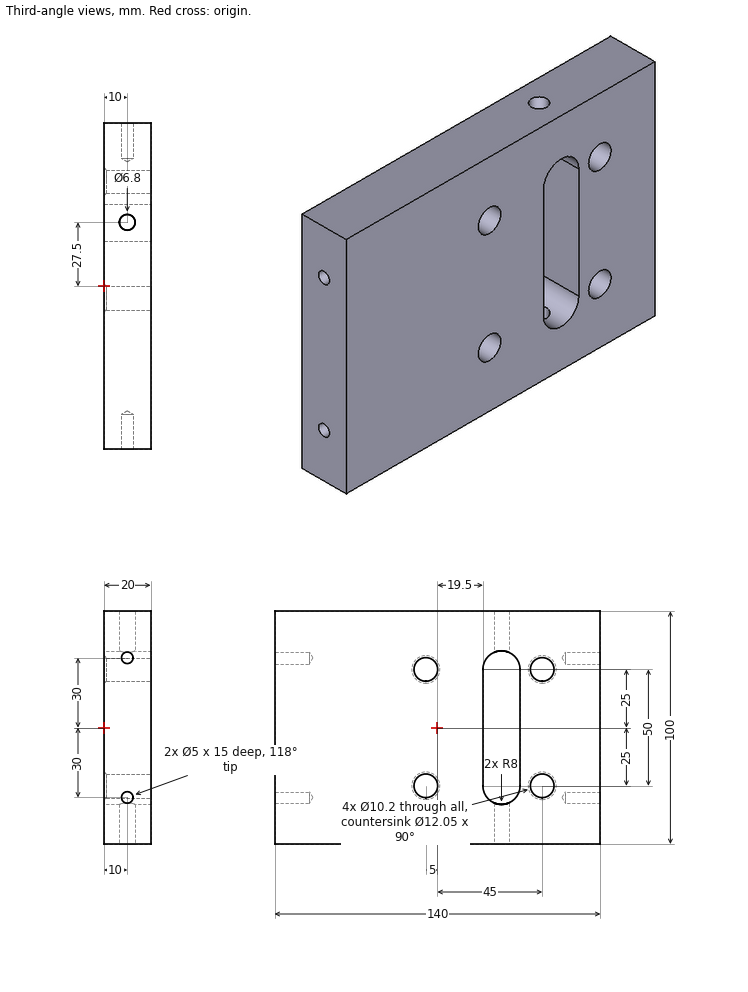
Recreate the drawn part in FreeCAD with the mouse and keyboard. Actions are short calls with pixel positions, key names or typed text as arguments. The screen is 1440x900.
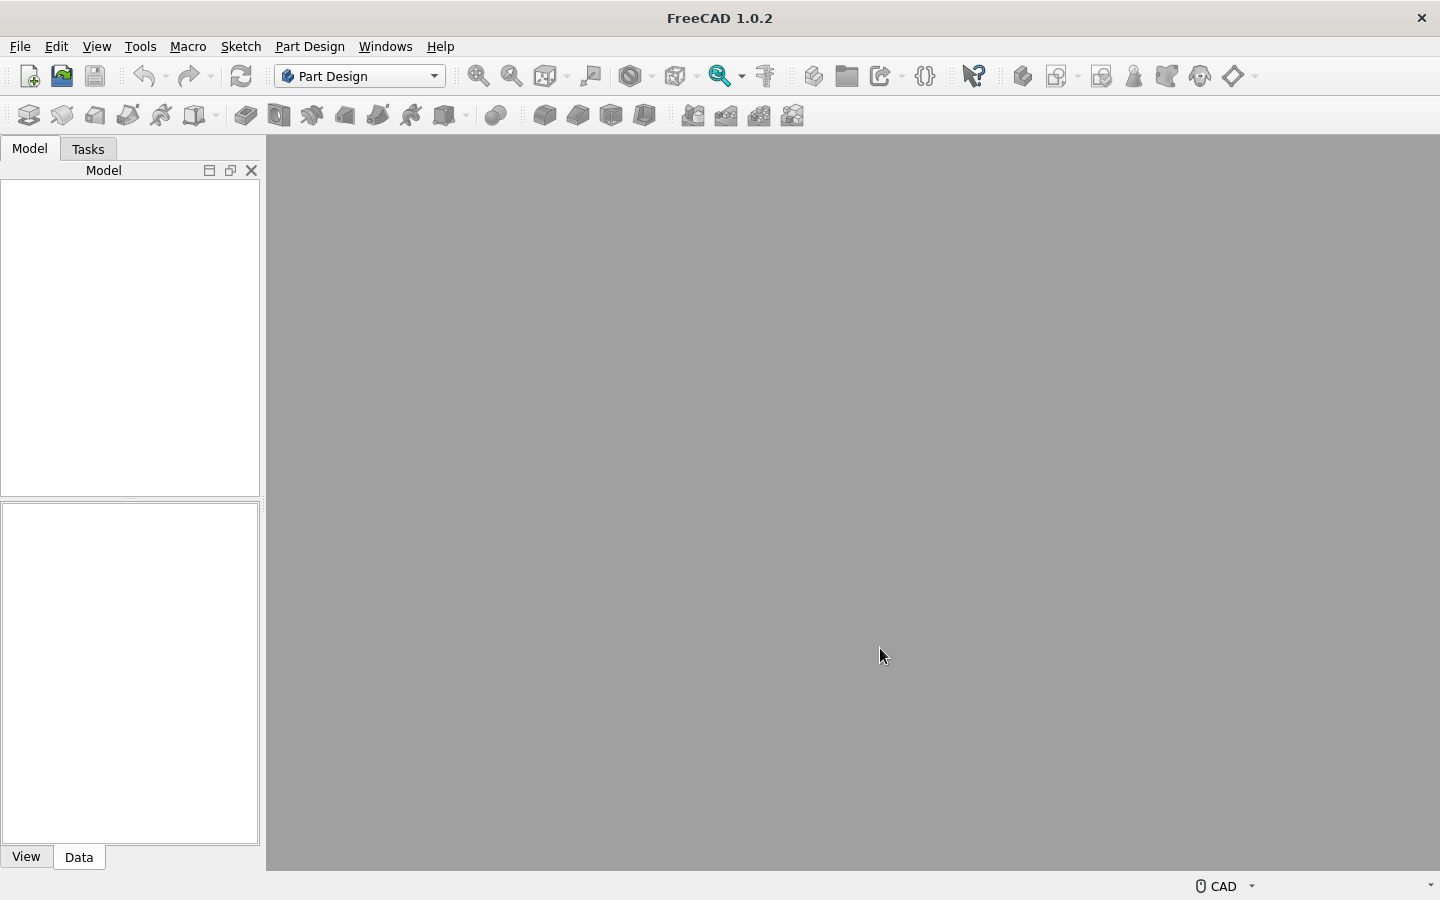
click(29, 76)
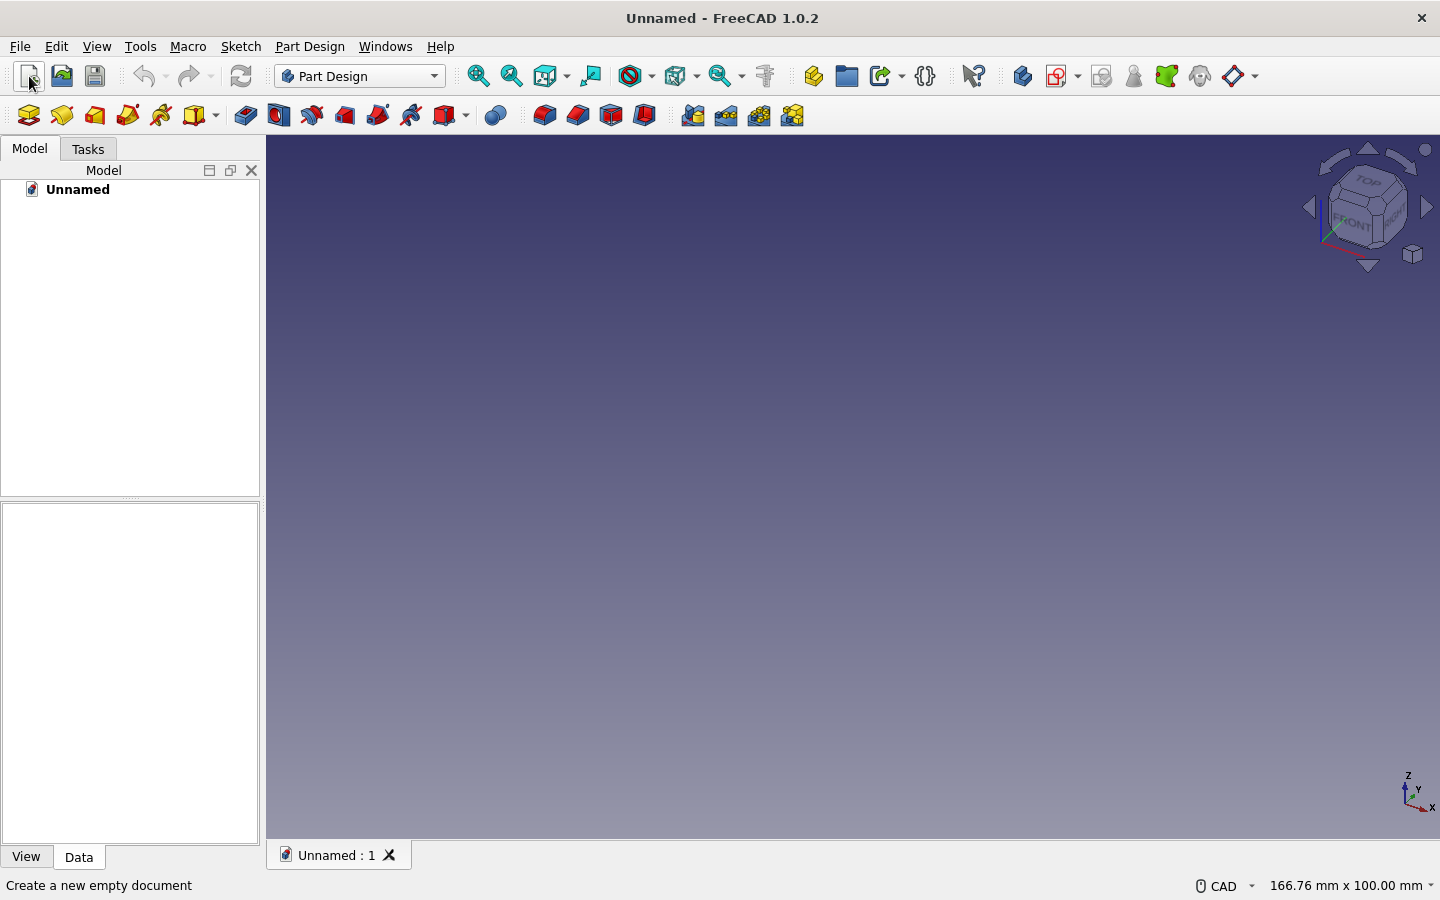
click(1056, 76)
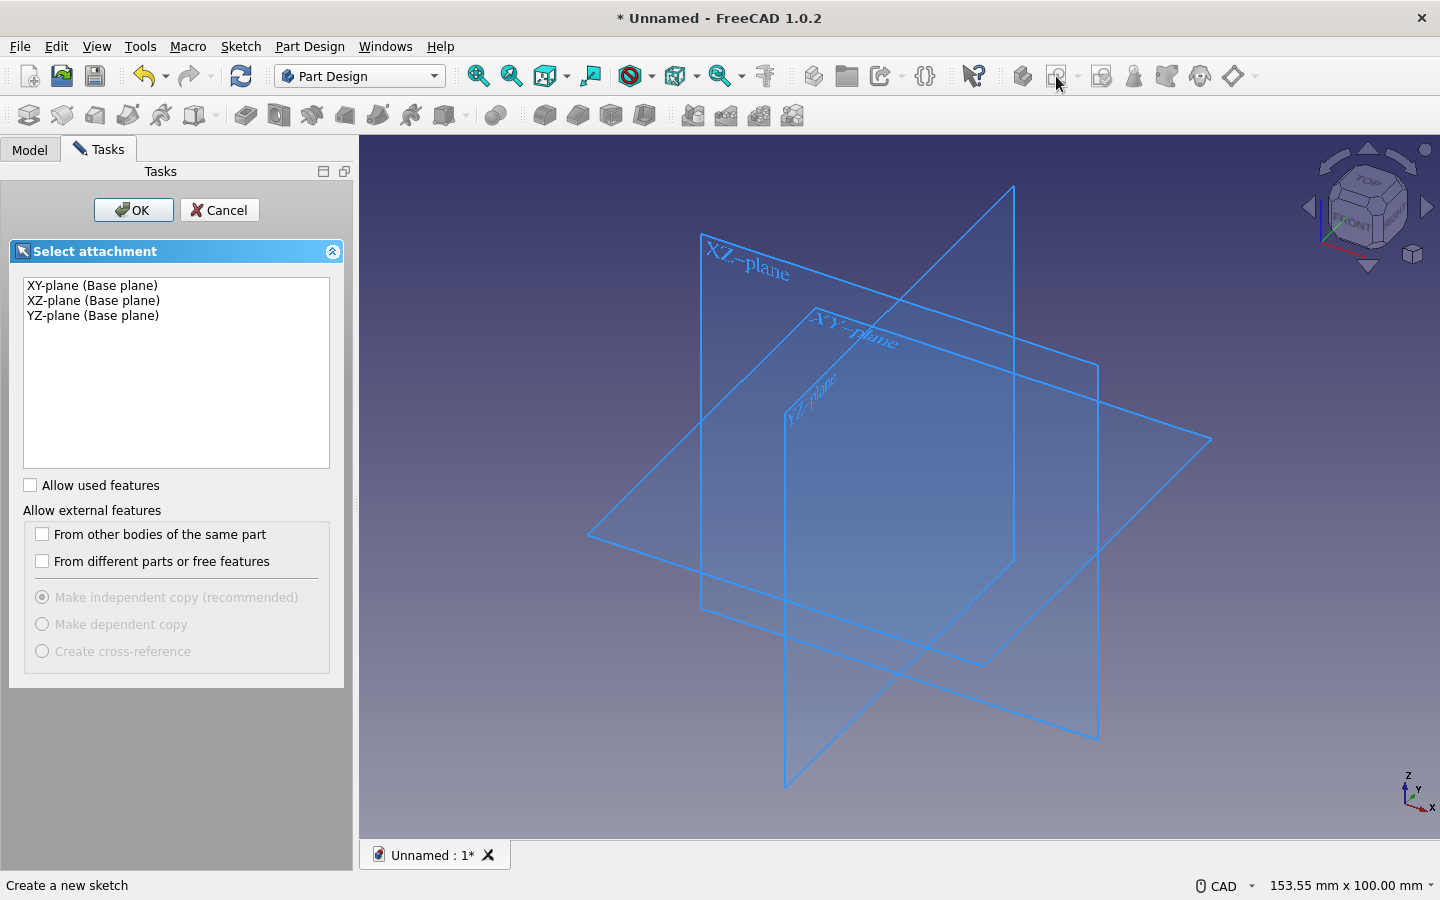
click(84, 316)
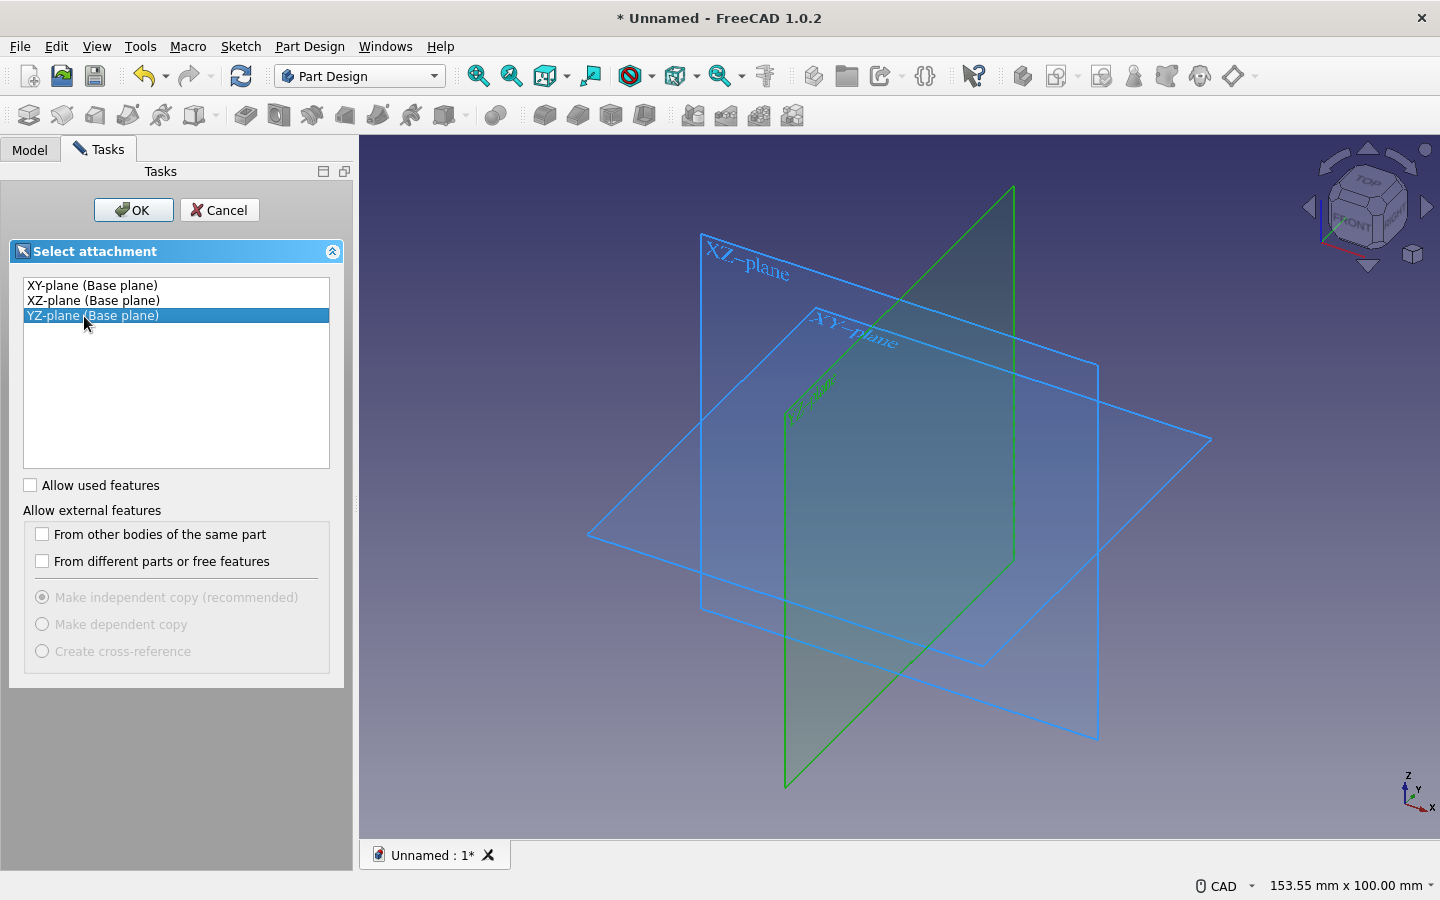
click(134, 210)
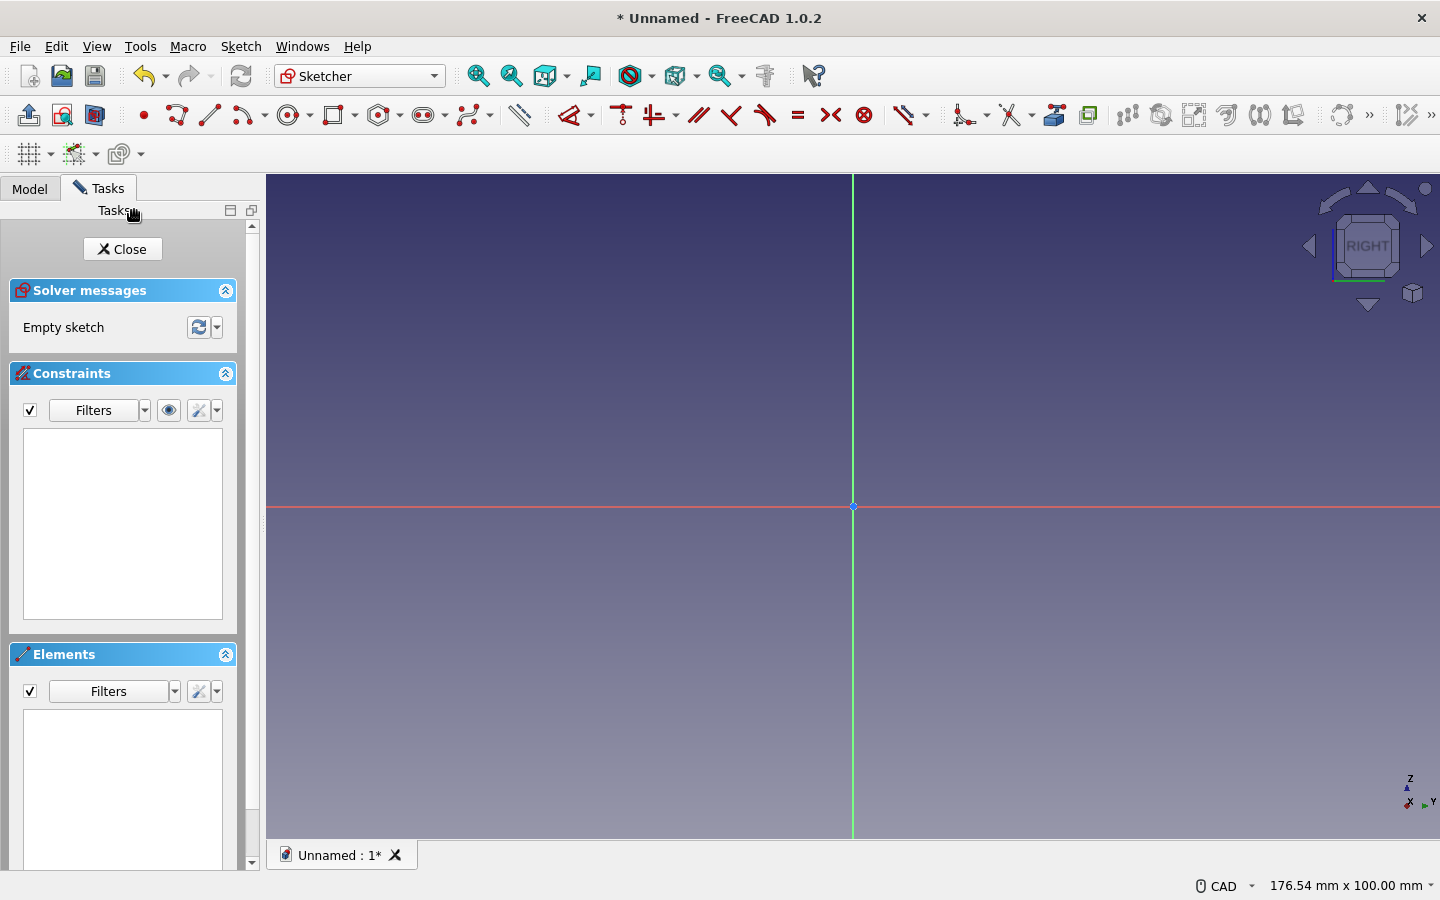
scroll(645, 507, down, 2)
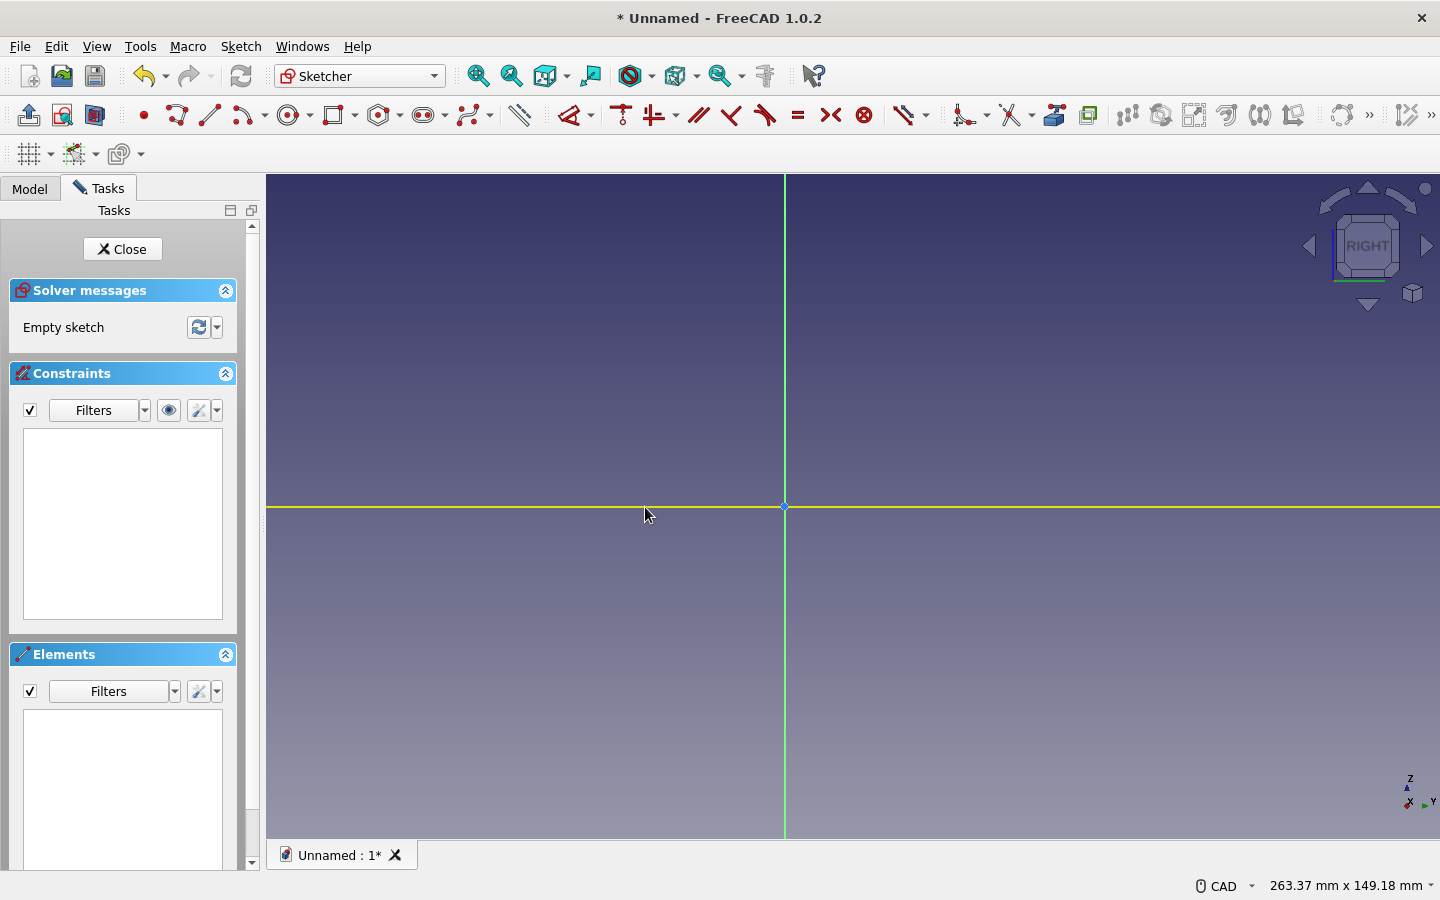
click(354, 116)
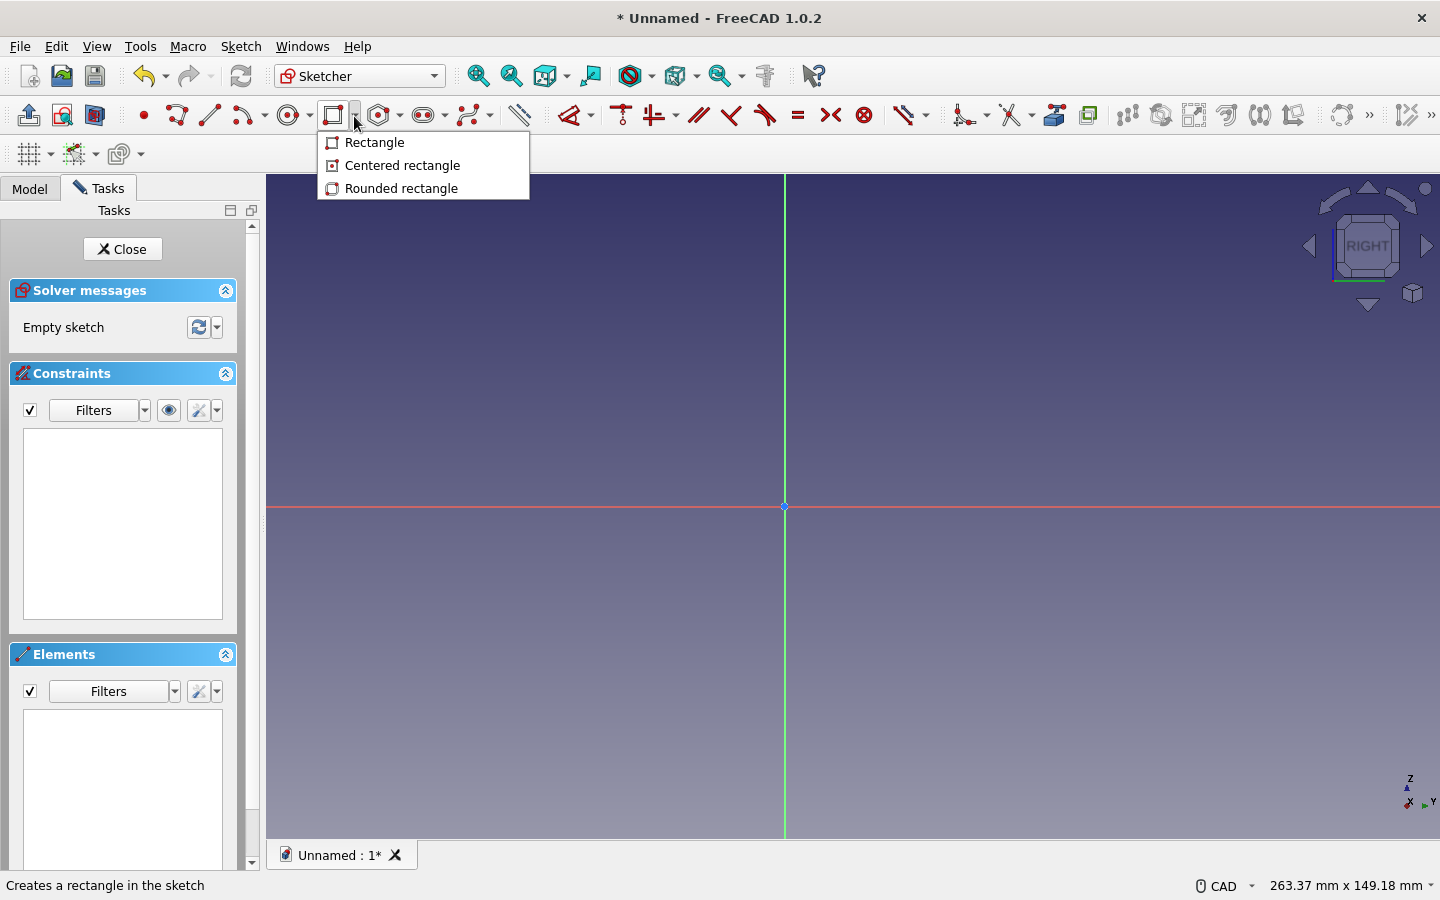
click(424, 166)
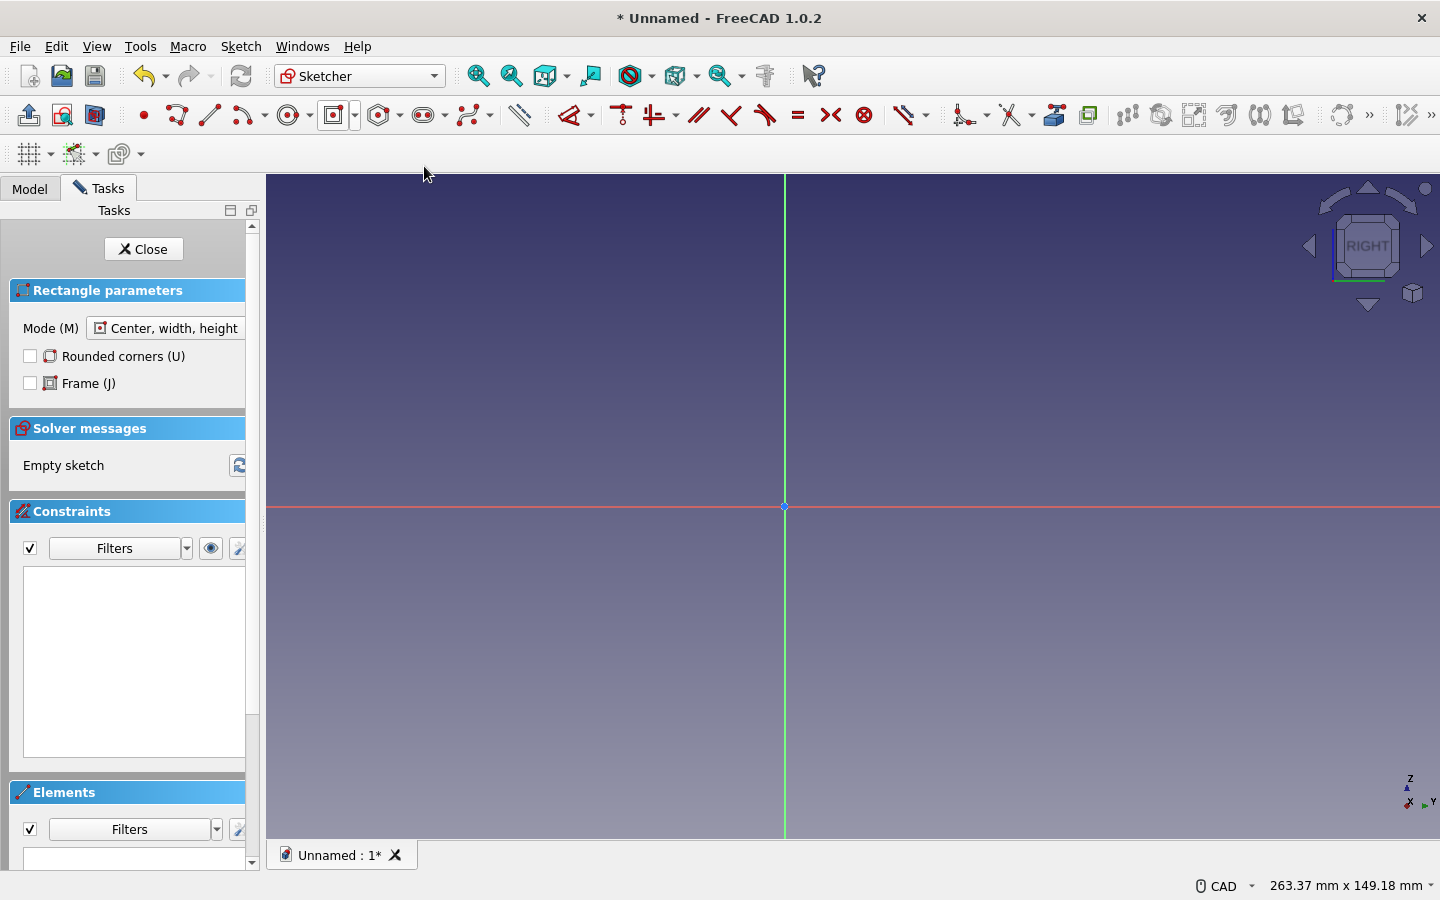
click(785, 507)
move(1097, 284)